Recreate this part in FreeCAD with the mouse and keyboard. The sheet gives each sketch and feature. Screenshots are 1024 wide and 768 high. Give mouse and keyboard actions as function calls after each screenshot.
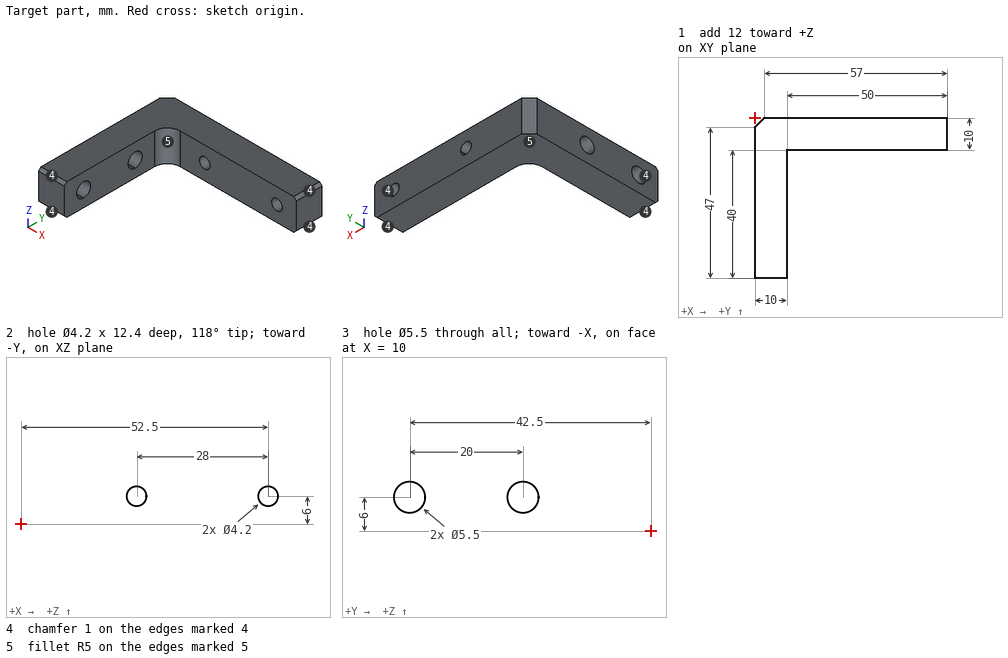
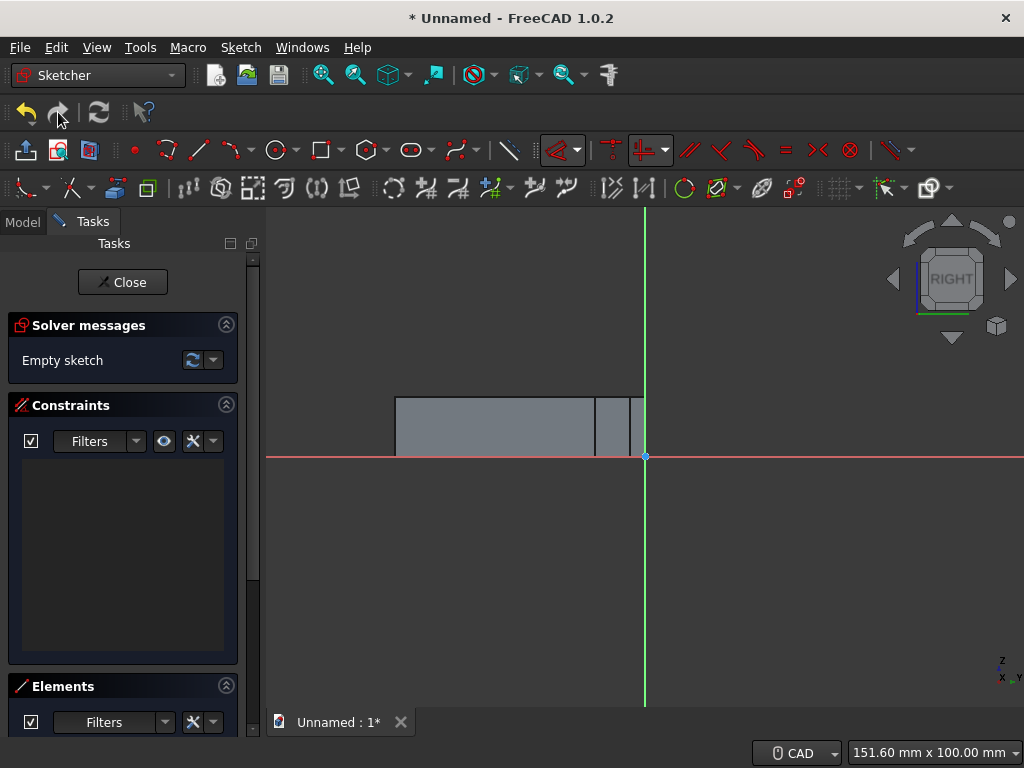
scroll(478, 409, up, 3)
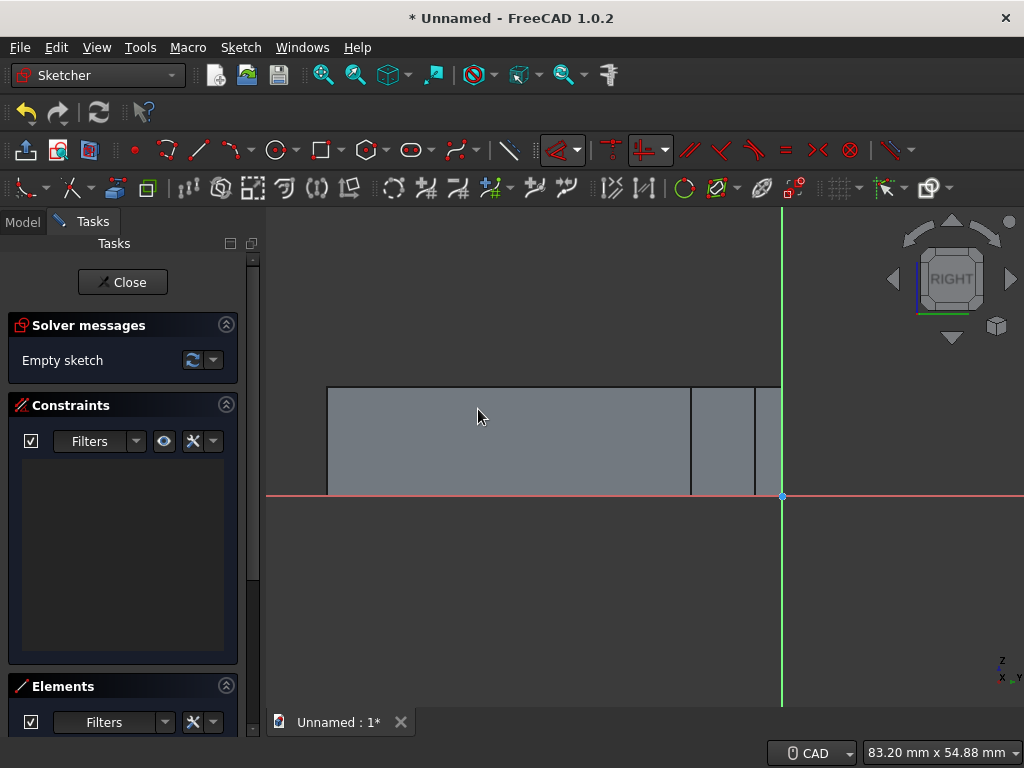
key(g)
key(c)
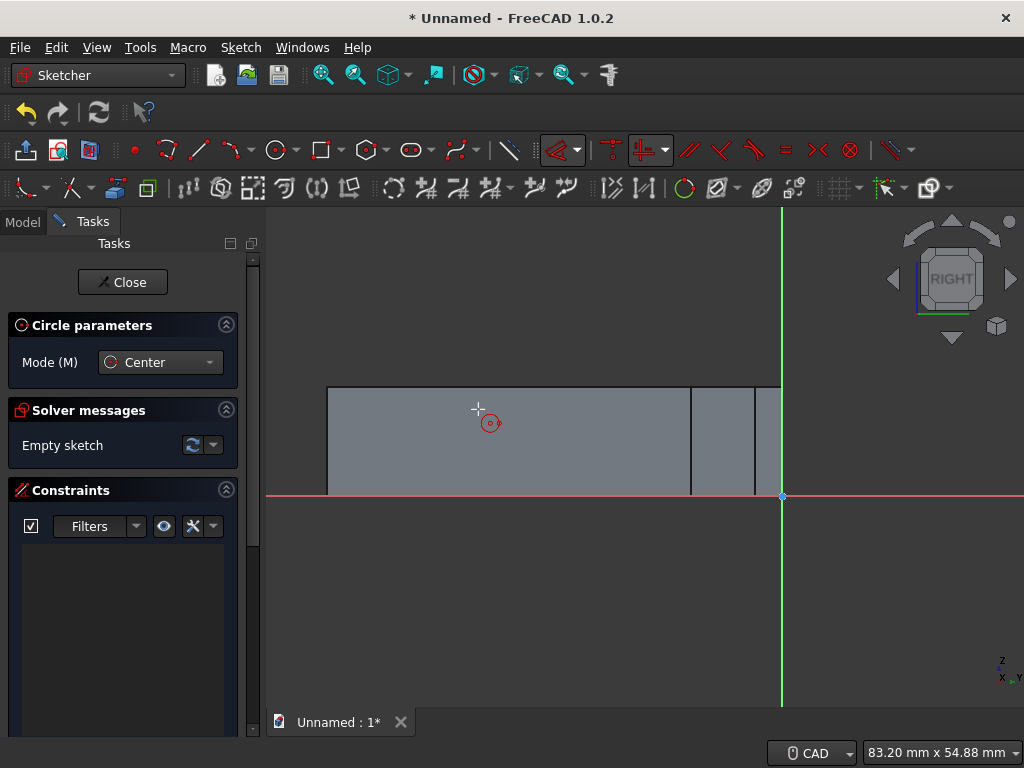
click(395, 441)
click(413, 424)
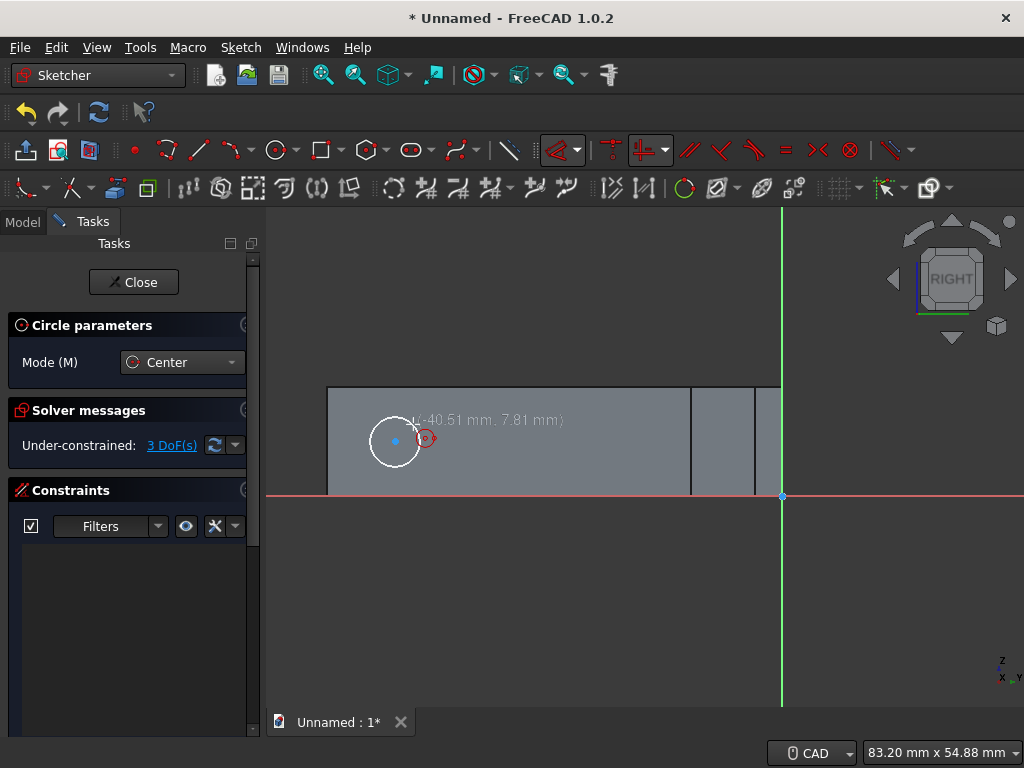
click(577, 441)
click(595, 424)
key(Escape)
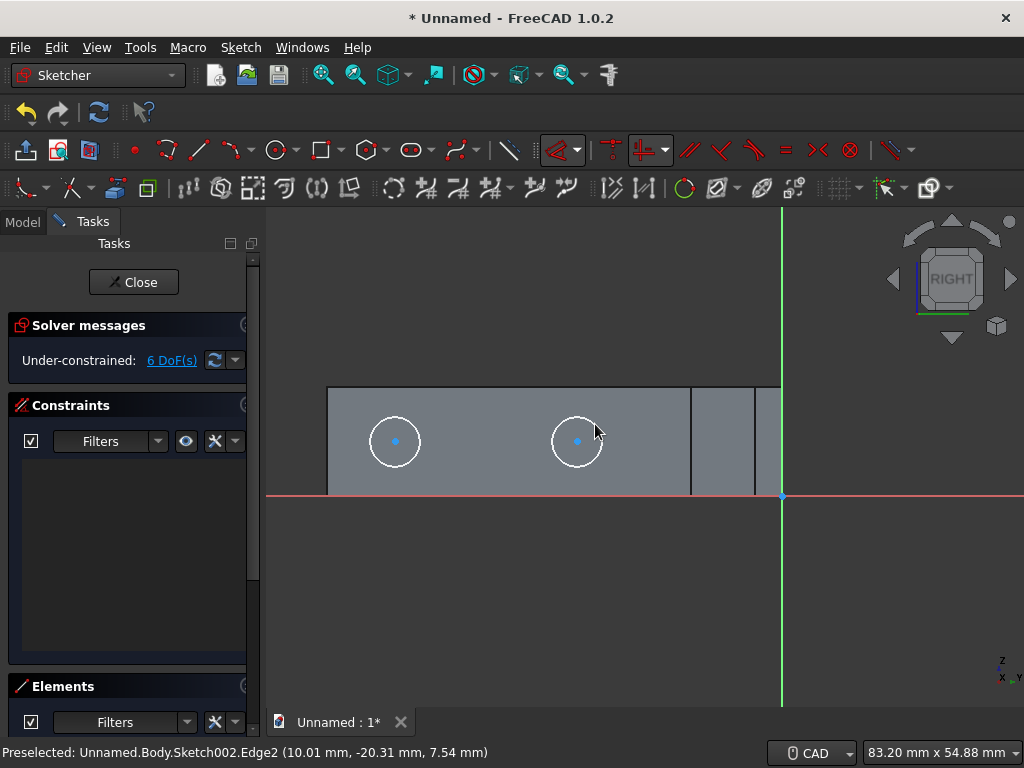
click(412, 424)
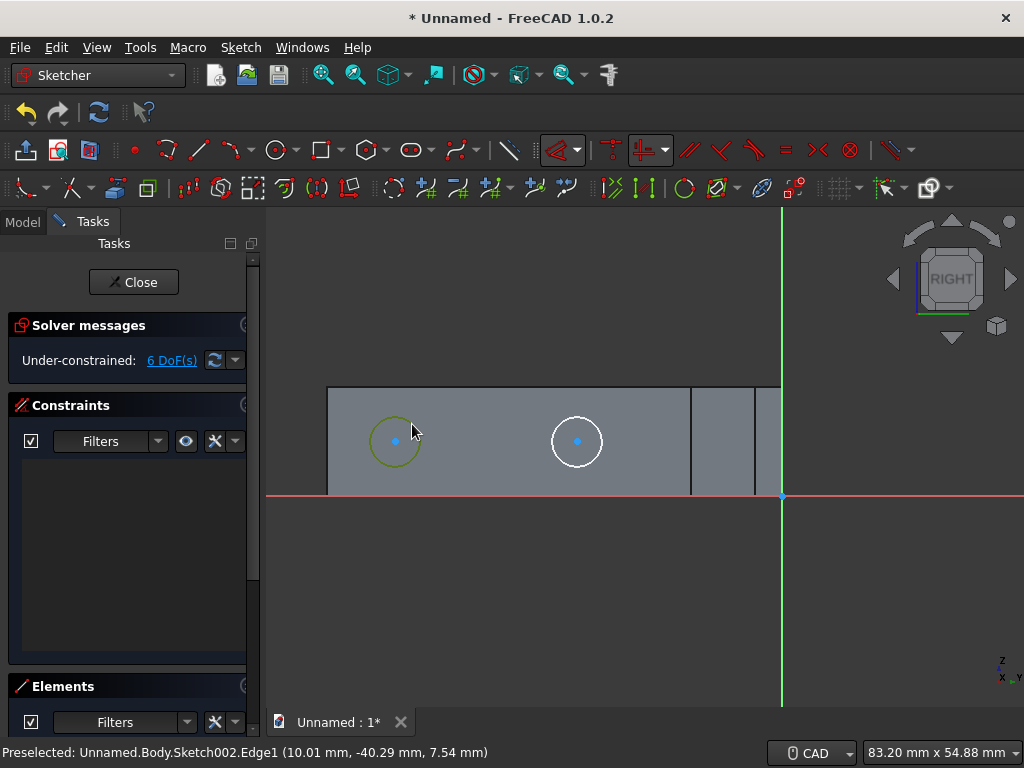
click(594, 424)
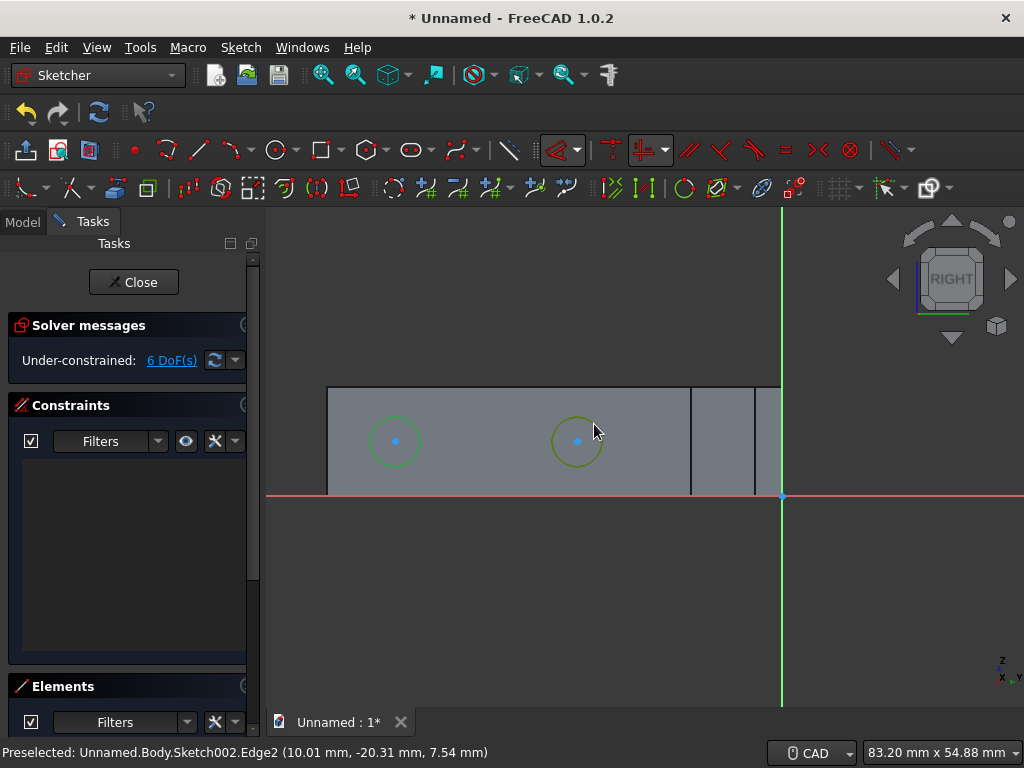
key(e)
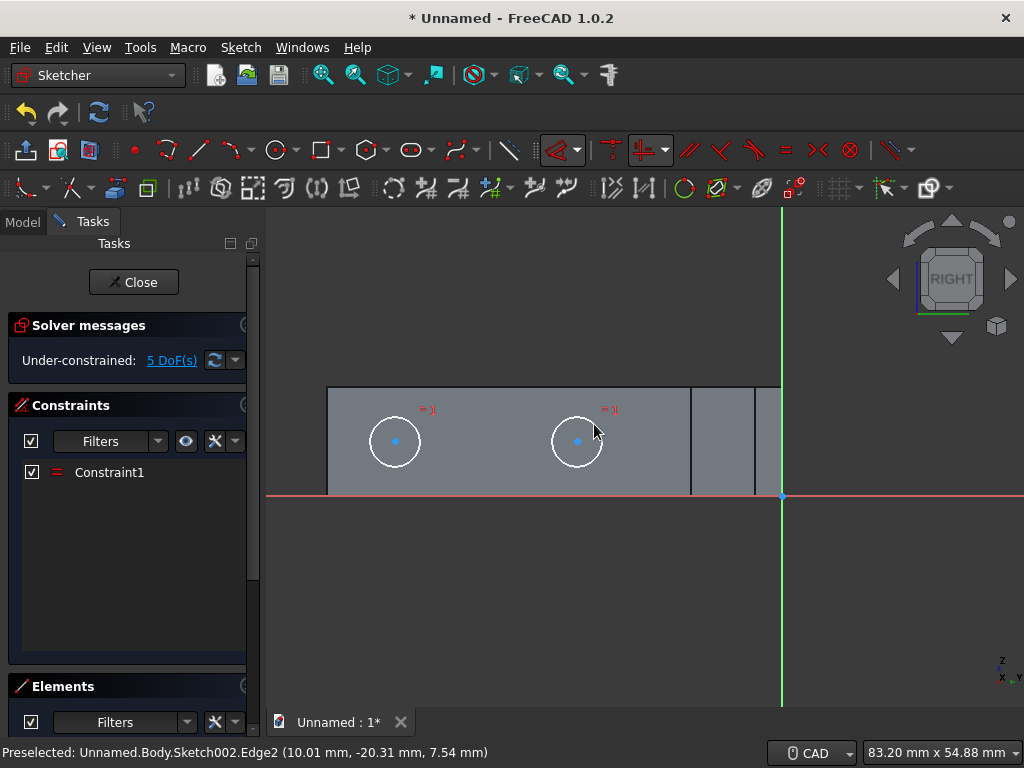
click(395, 442)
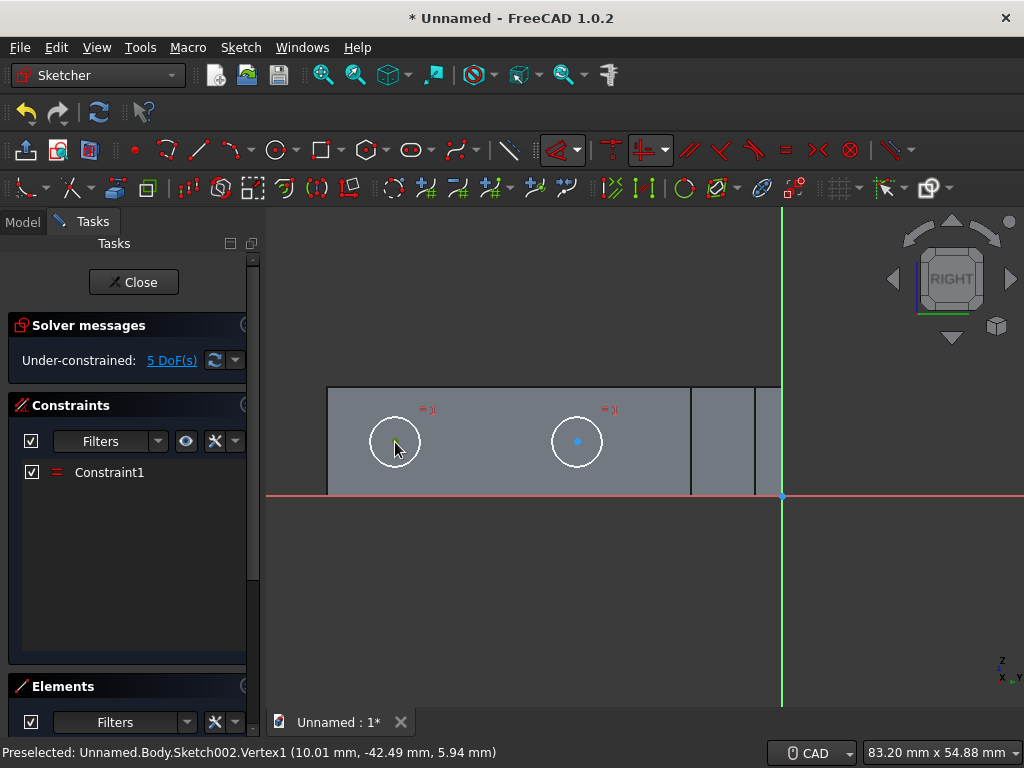
click(577, 442)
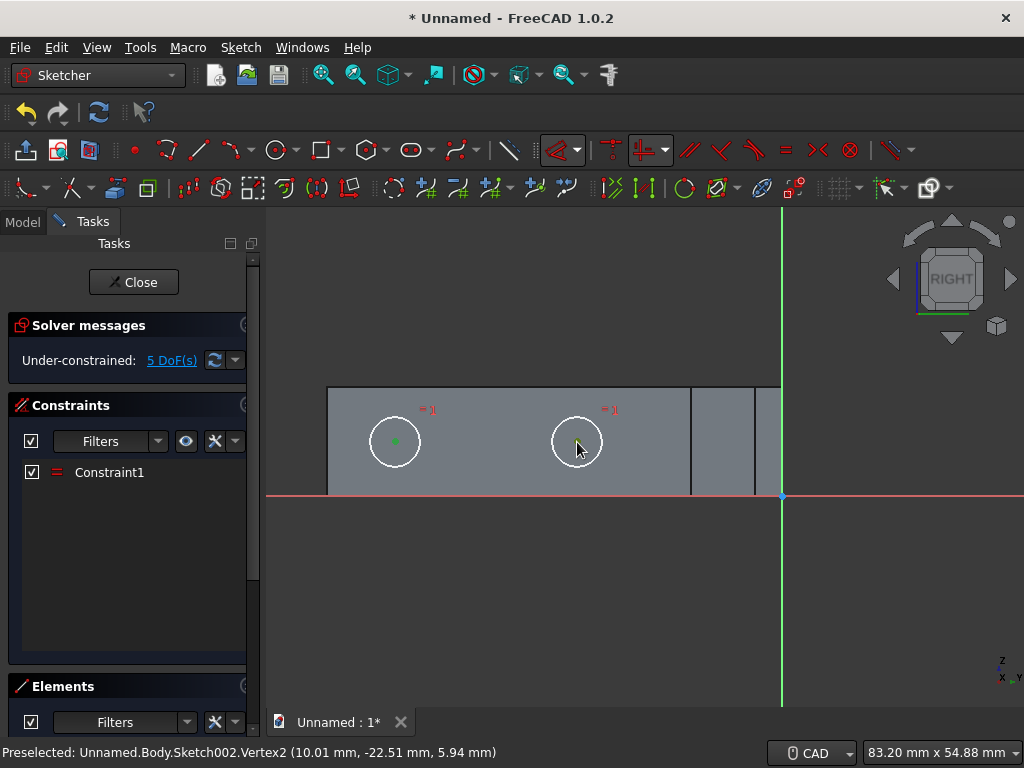
key(h)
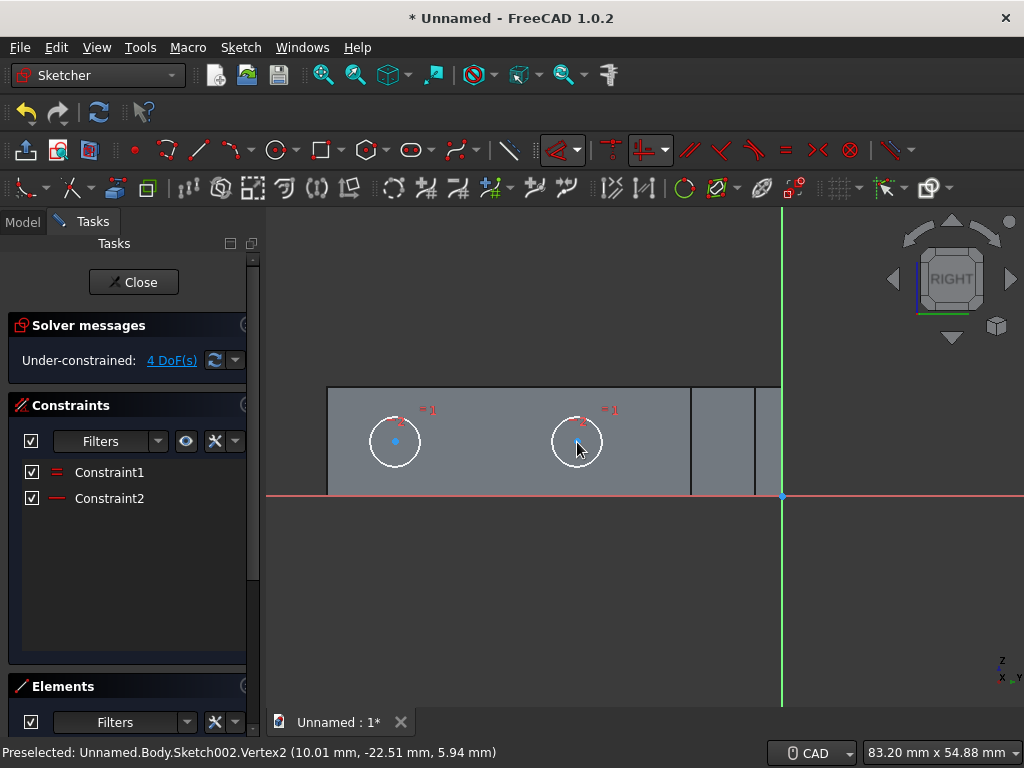
click(556, 150)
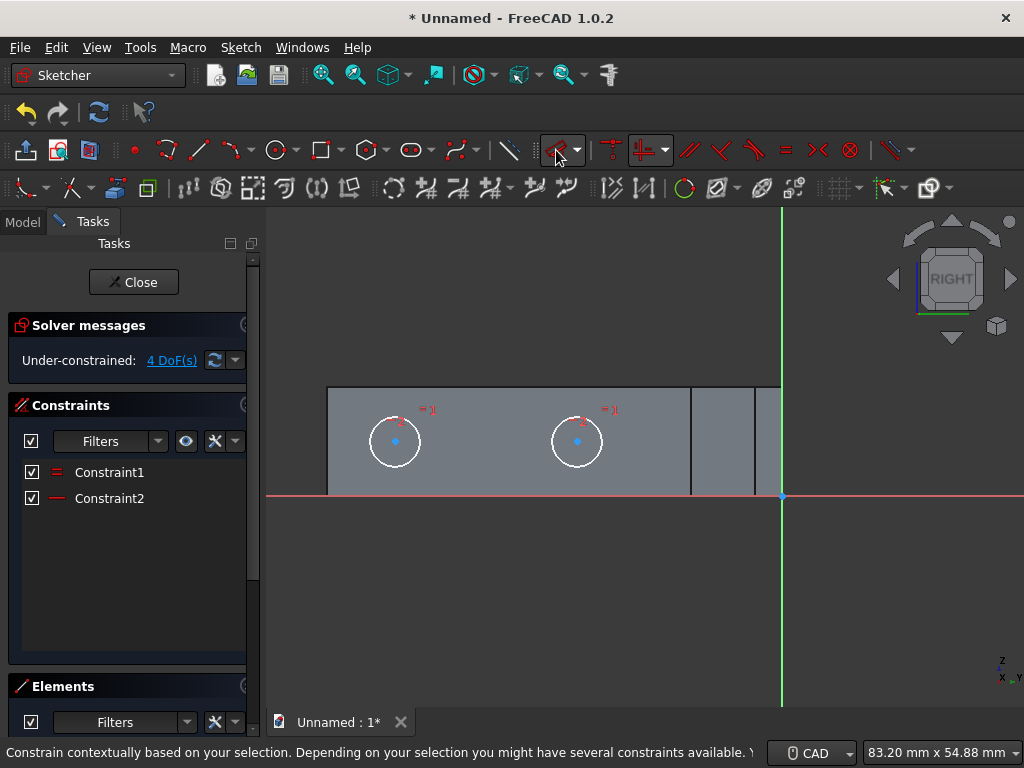
click(412, 424)
click(434, 401)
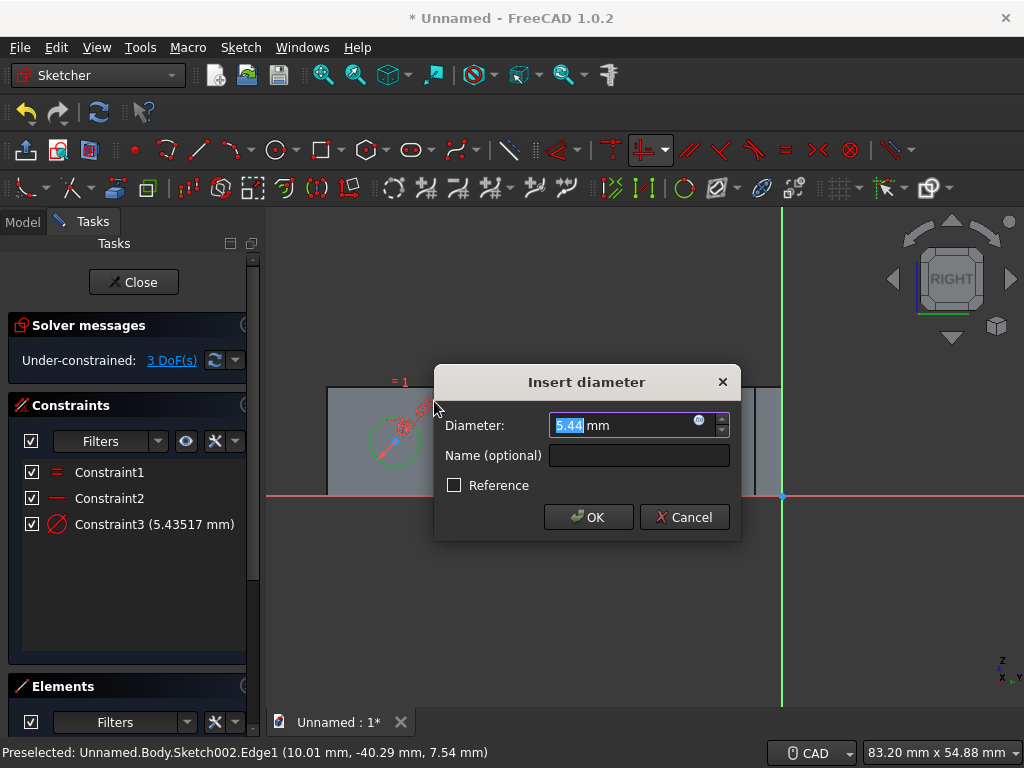
text(5.5)
key(Return)